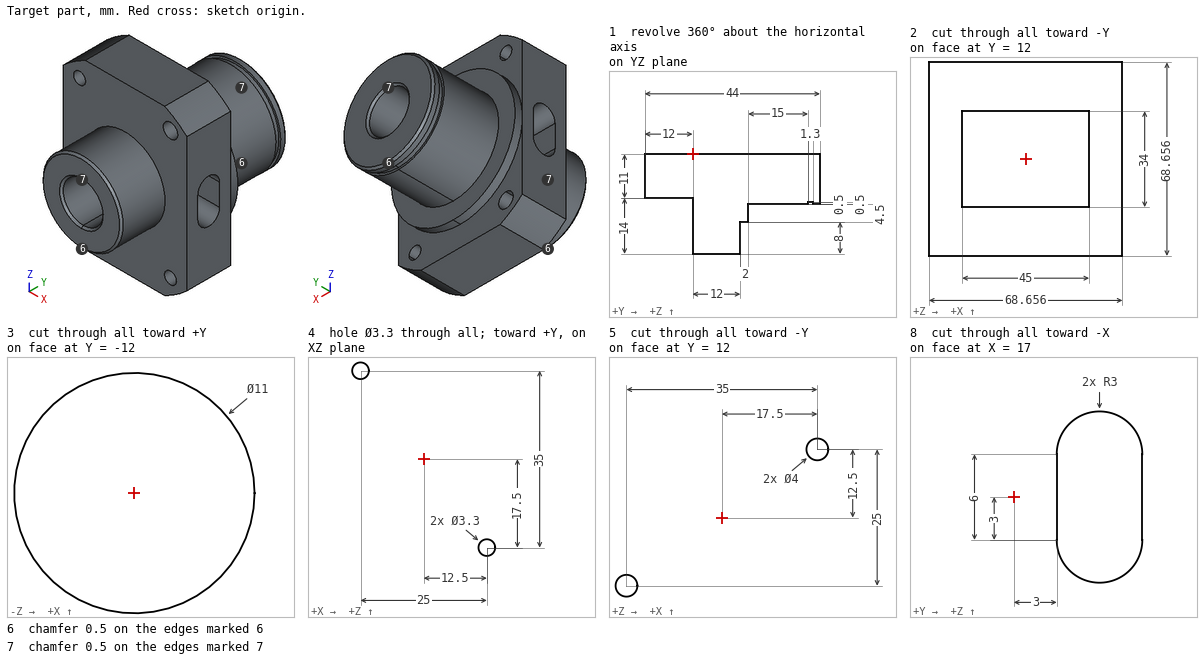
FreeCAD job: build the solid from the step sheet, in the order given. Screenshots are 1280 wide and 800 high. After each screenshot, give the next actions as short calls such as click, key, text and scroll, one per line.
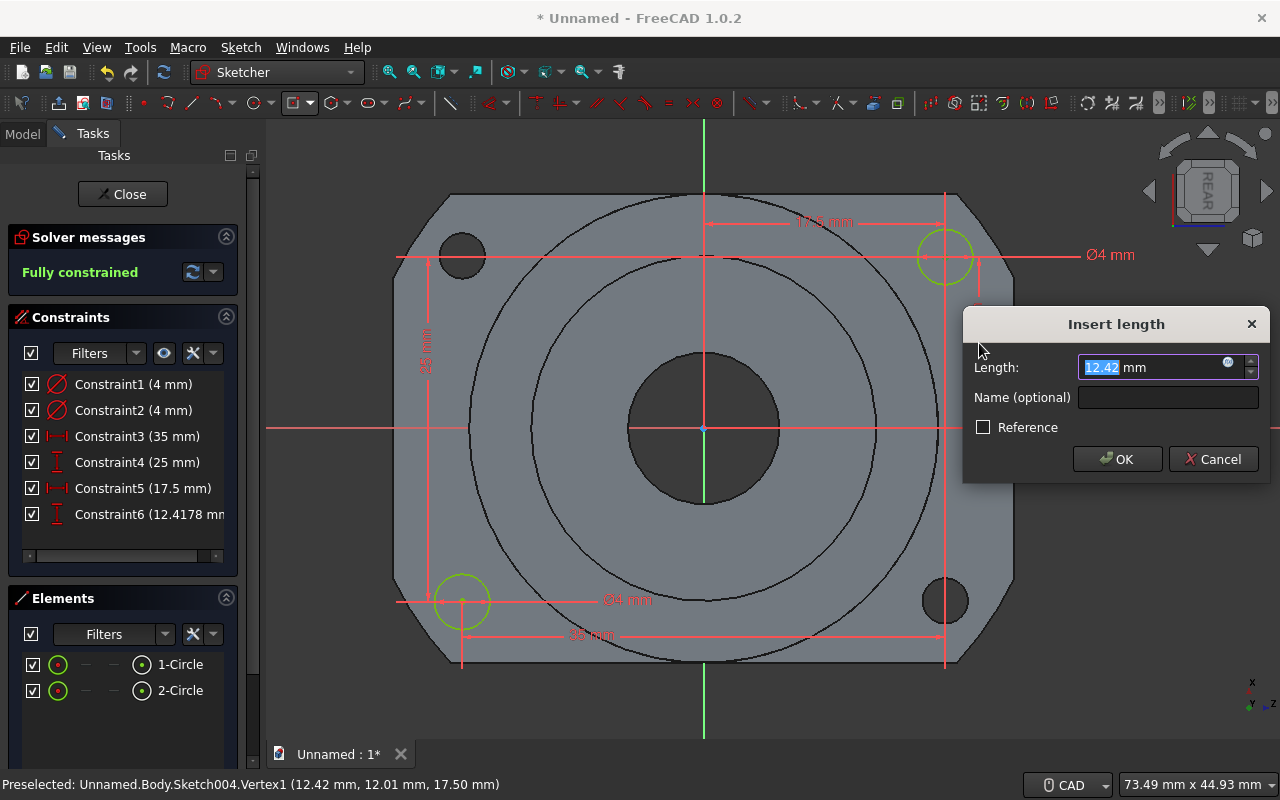
text(12.5)
key(Return)
key(Escape)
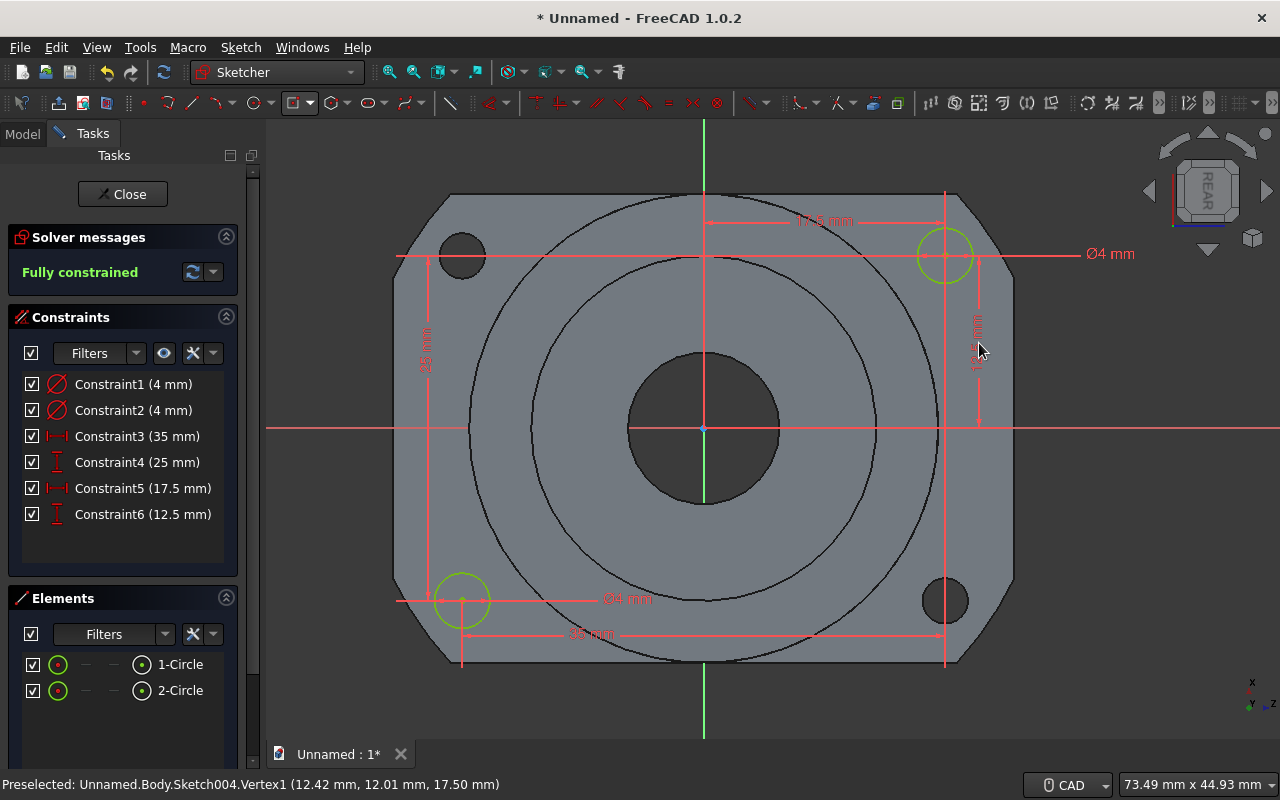
click(123, 194)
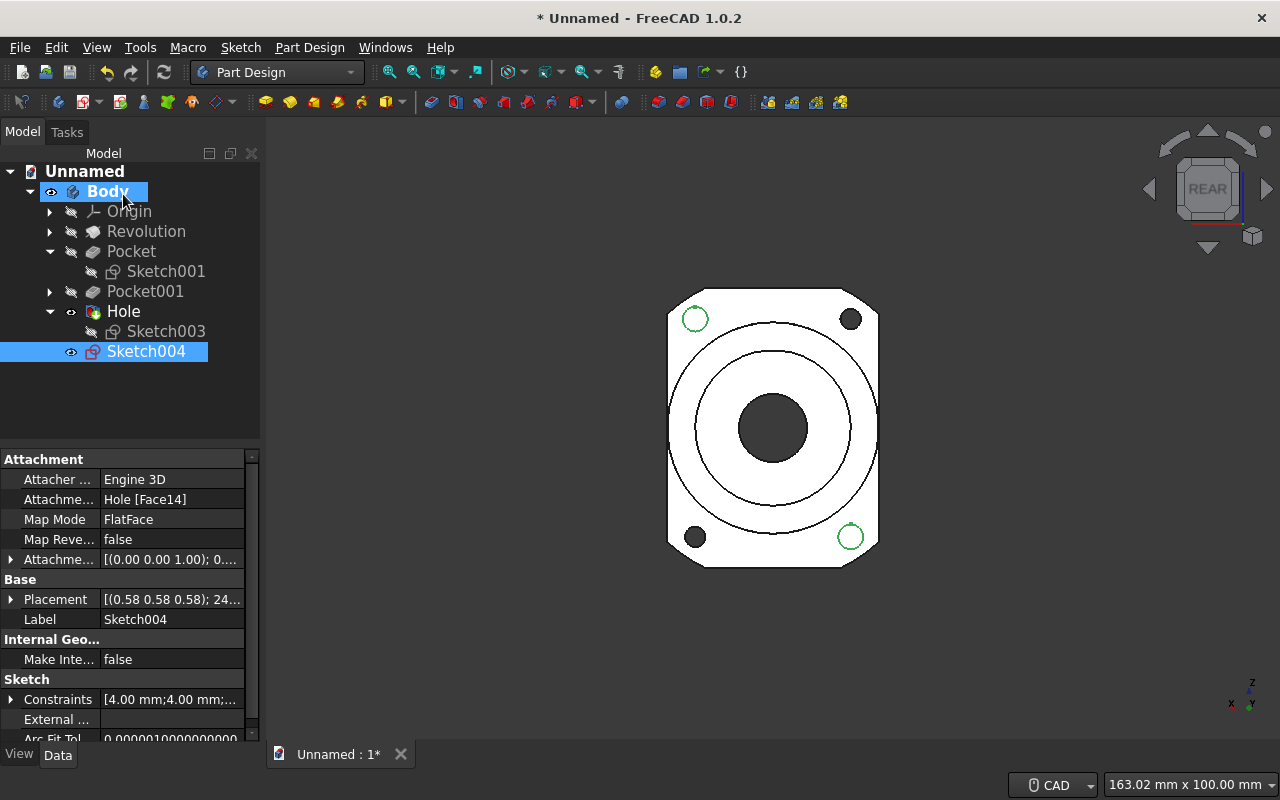
click(432, 102)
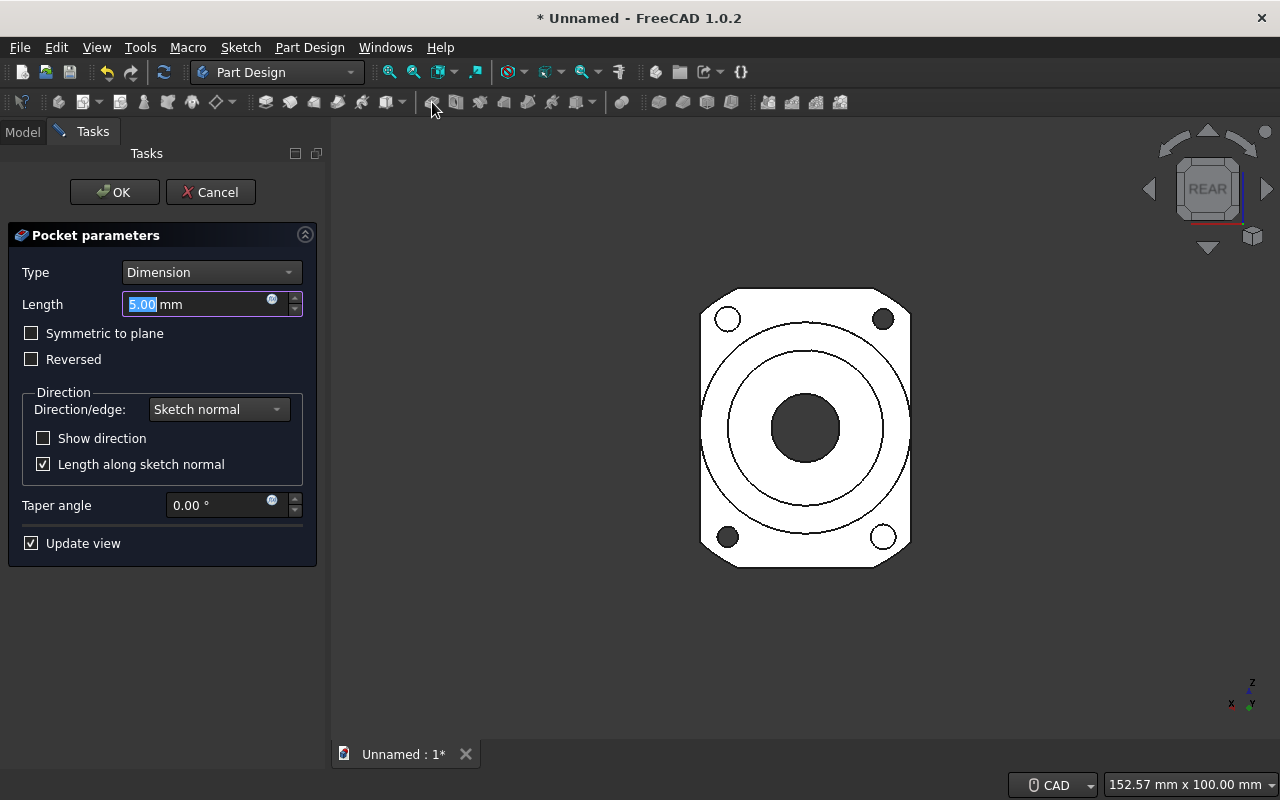
click(212, 272)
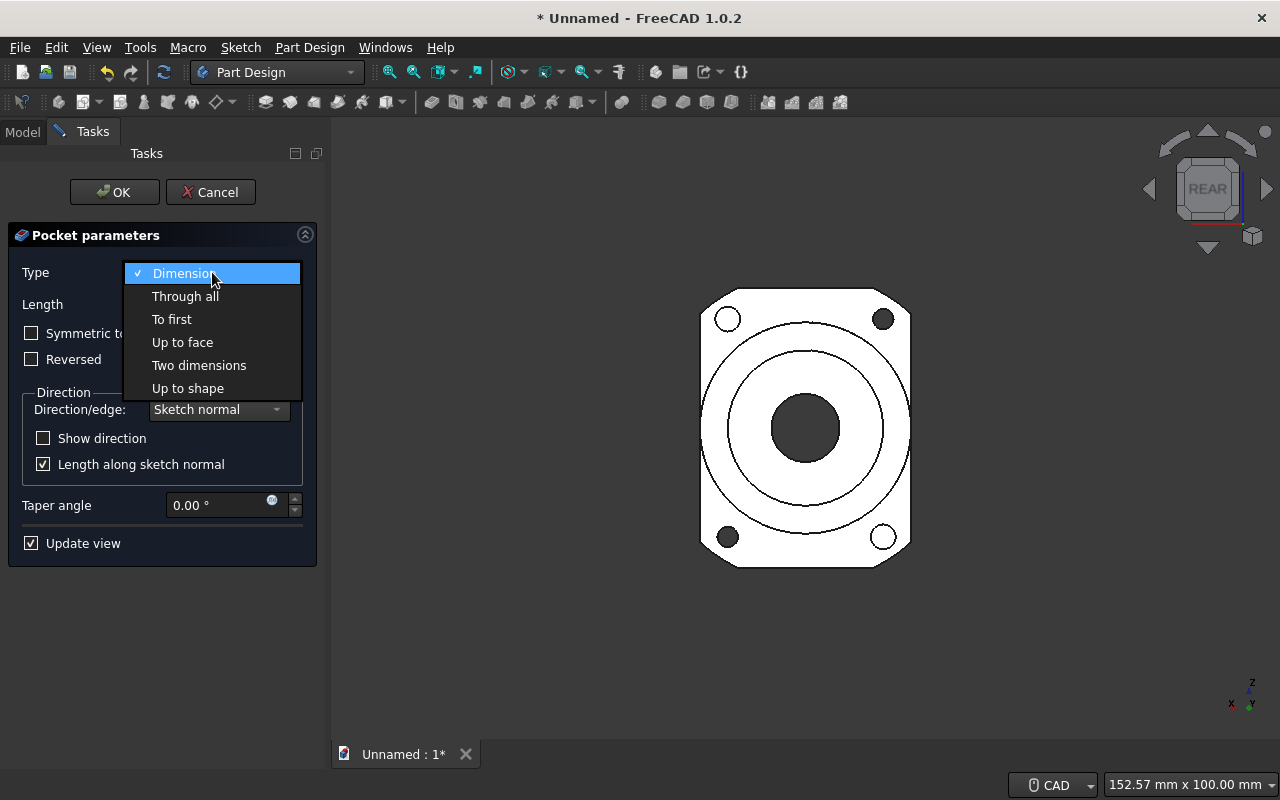
click(212, 296)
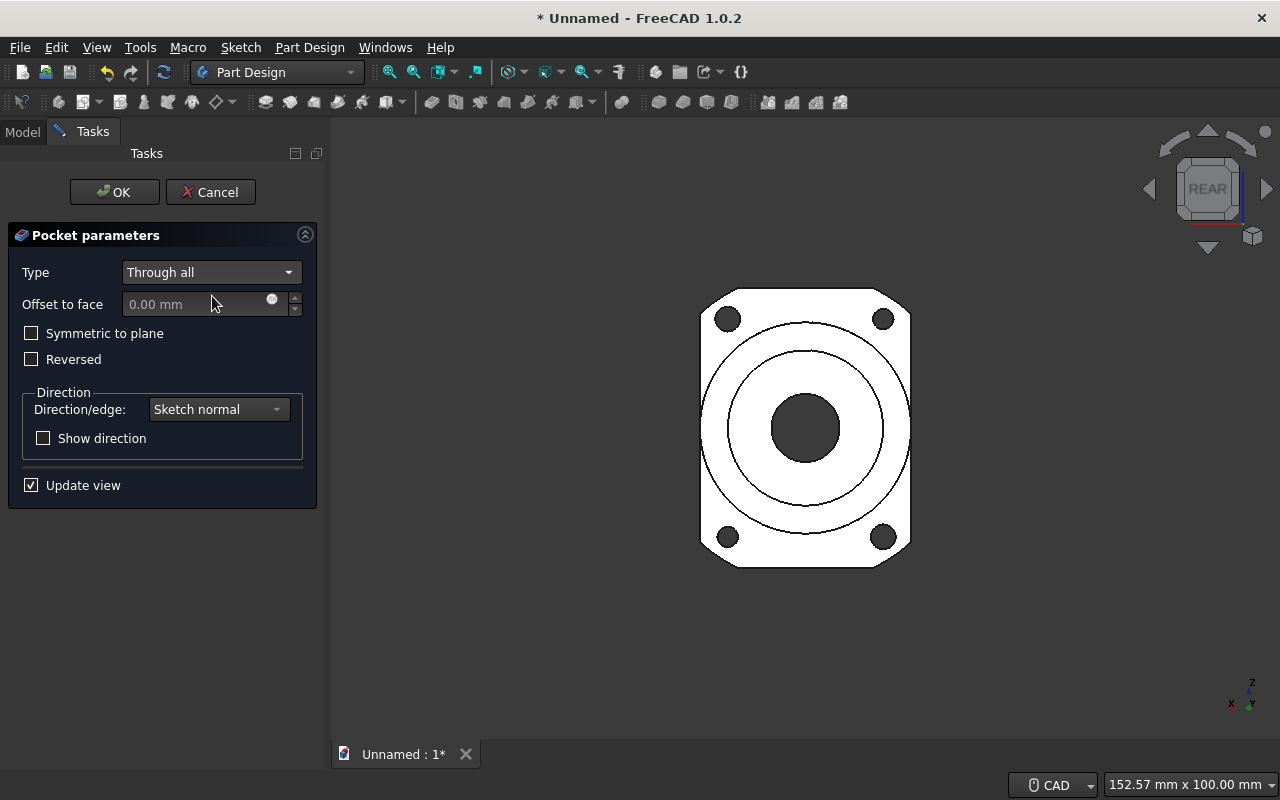
click(115, 192)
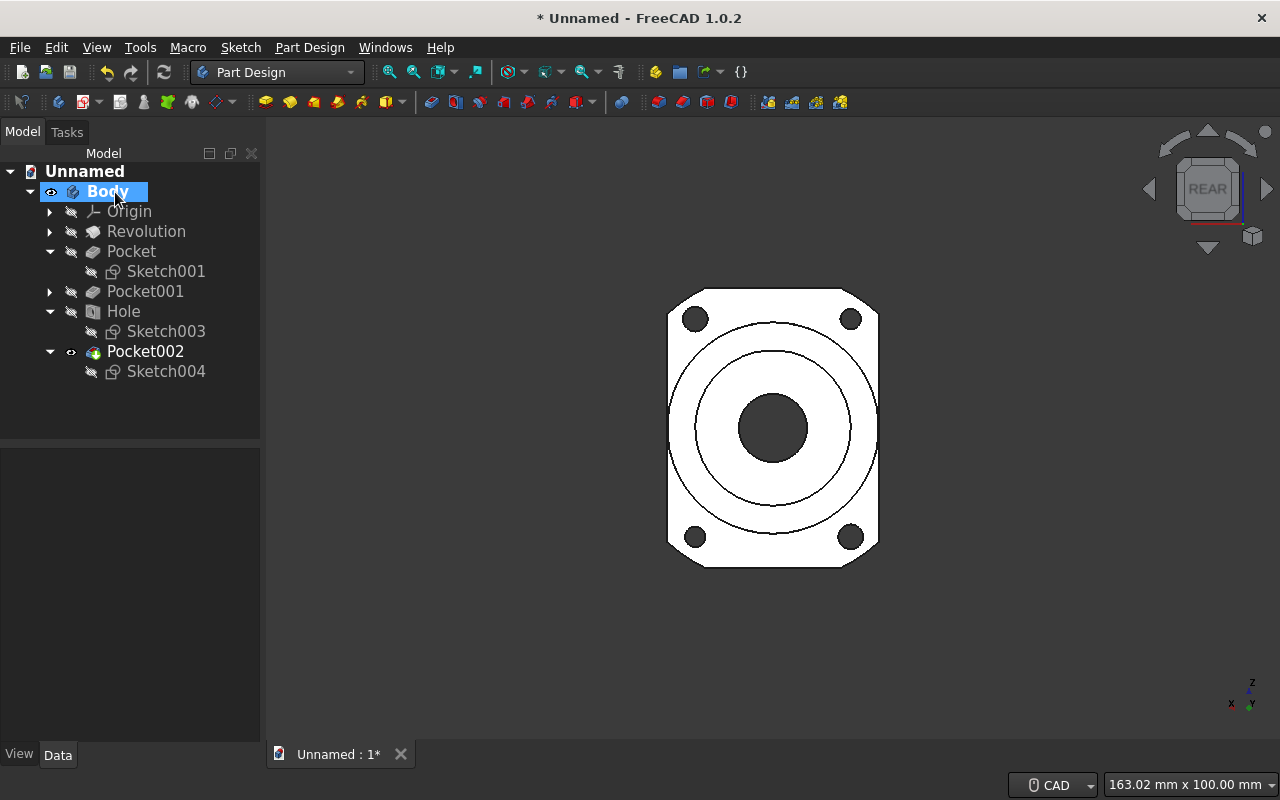
click(773, 349)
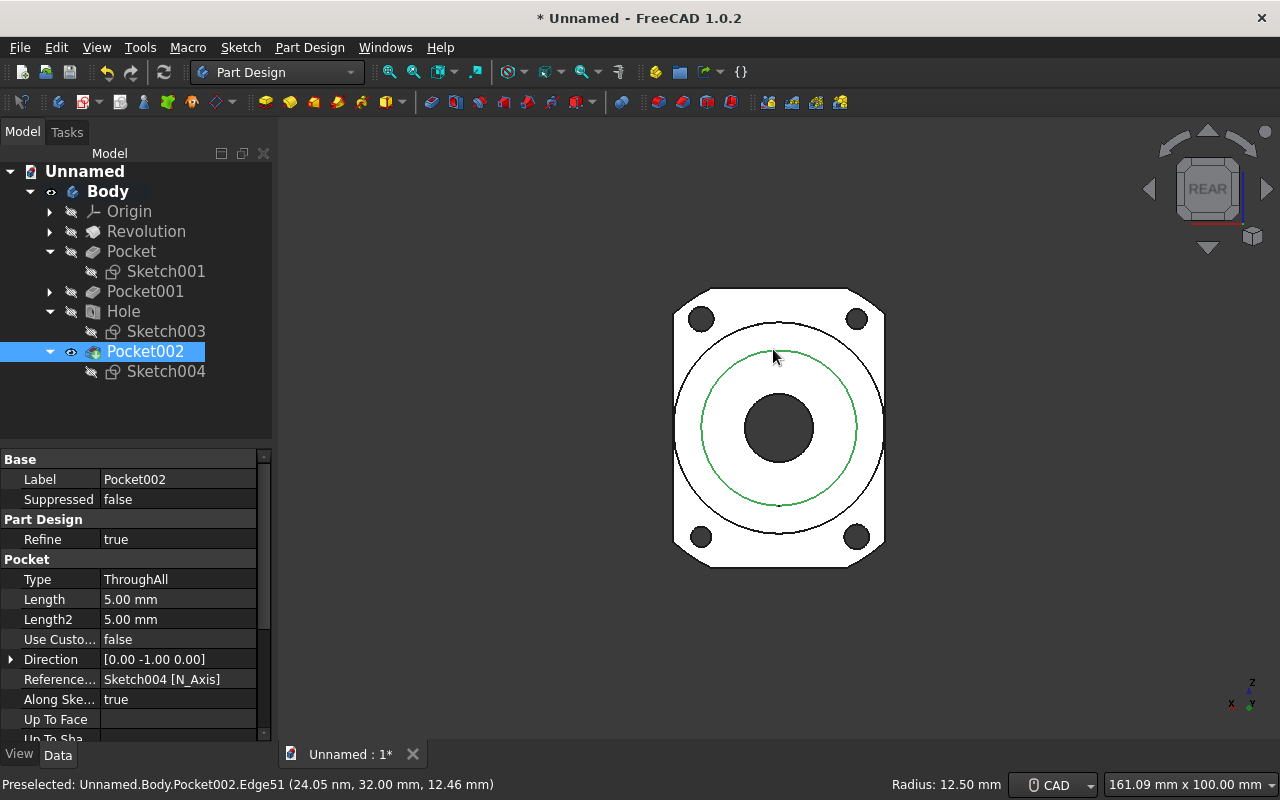
key(0)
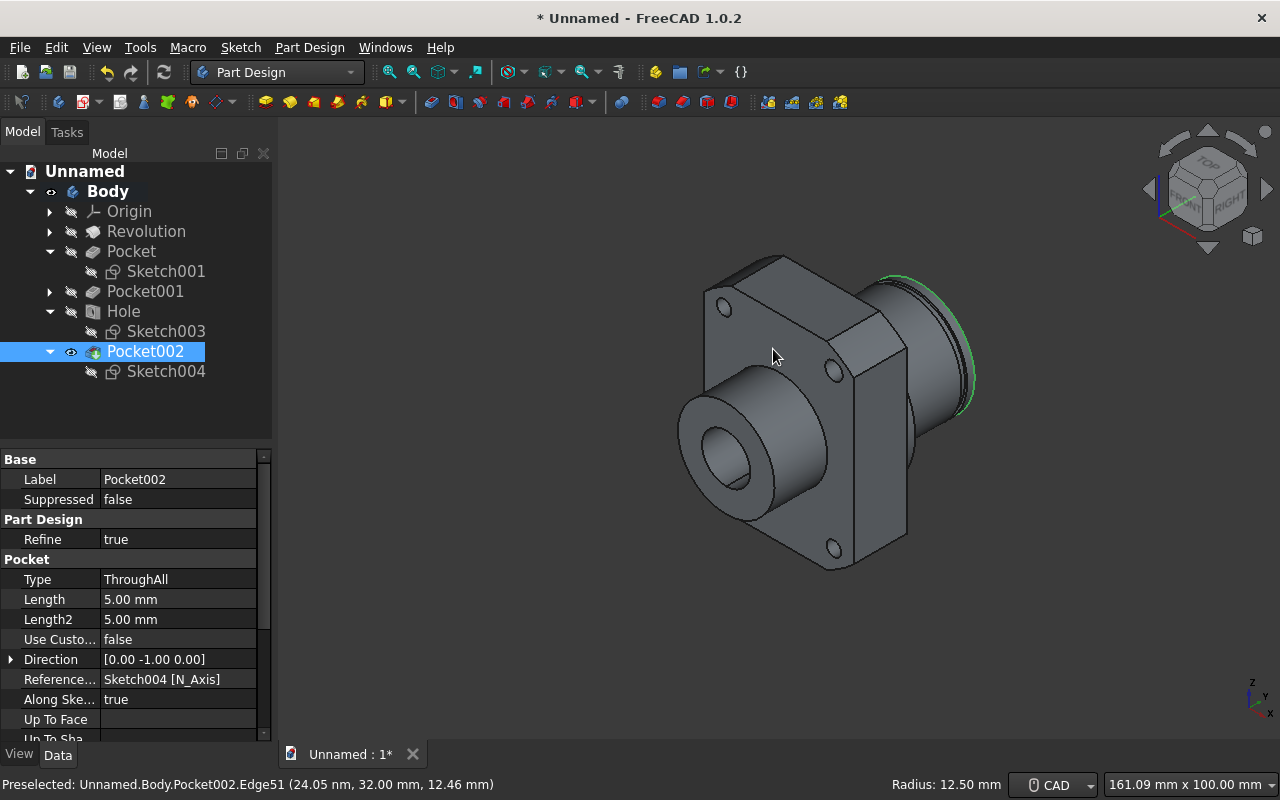
click(726, 402, ctrl)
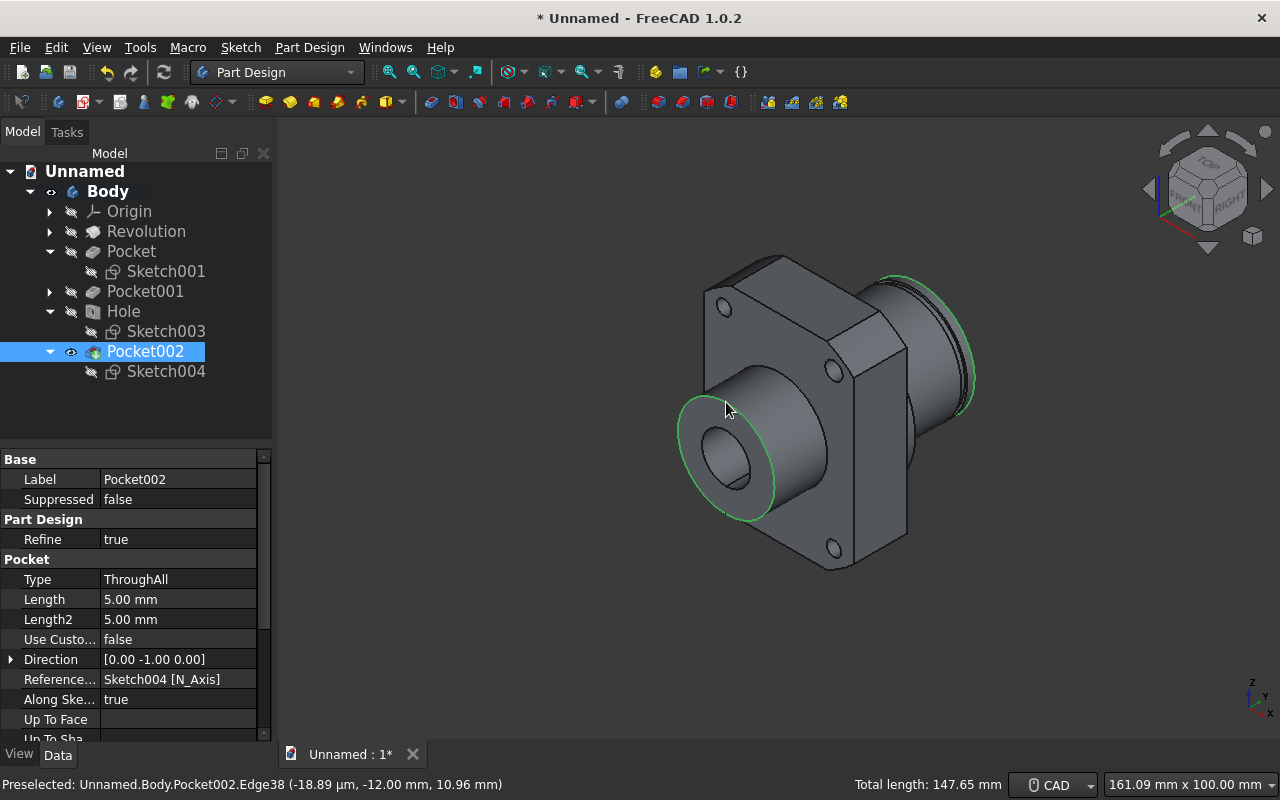
click(684, 102)